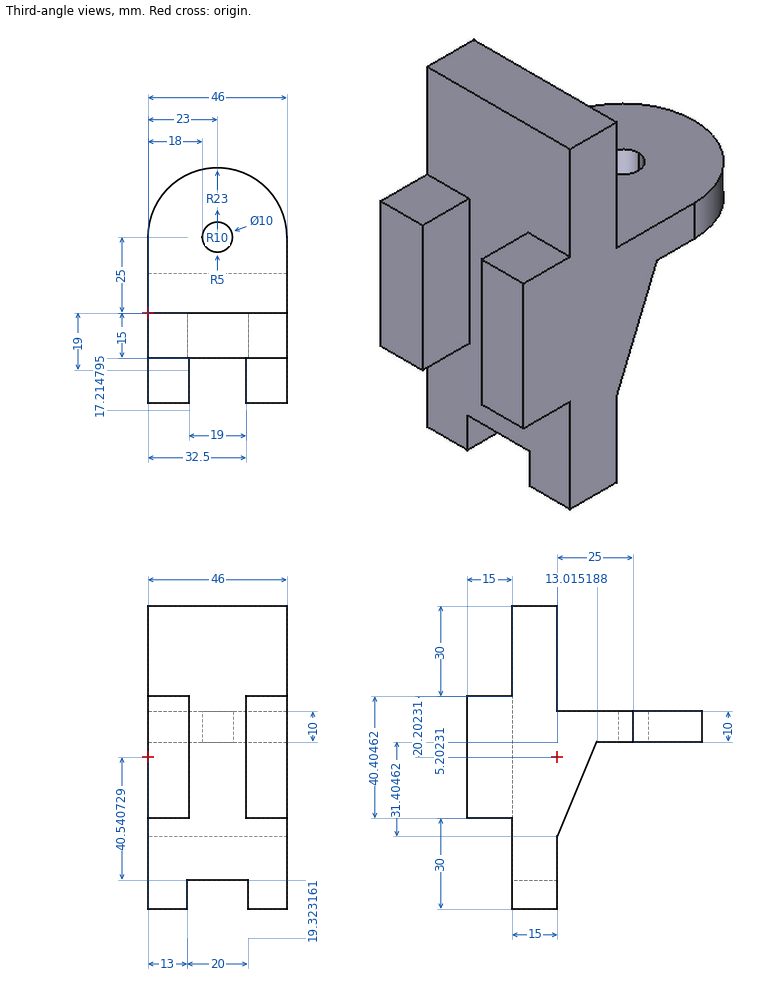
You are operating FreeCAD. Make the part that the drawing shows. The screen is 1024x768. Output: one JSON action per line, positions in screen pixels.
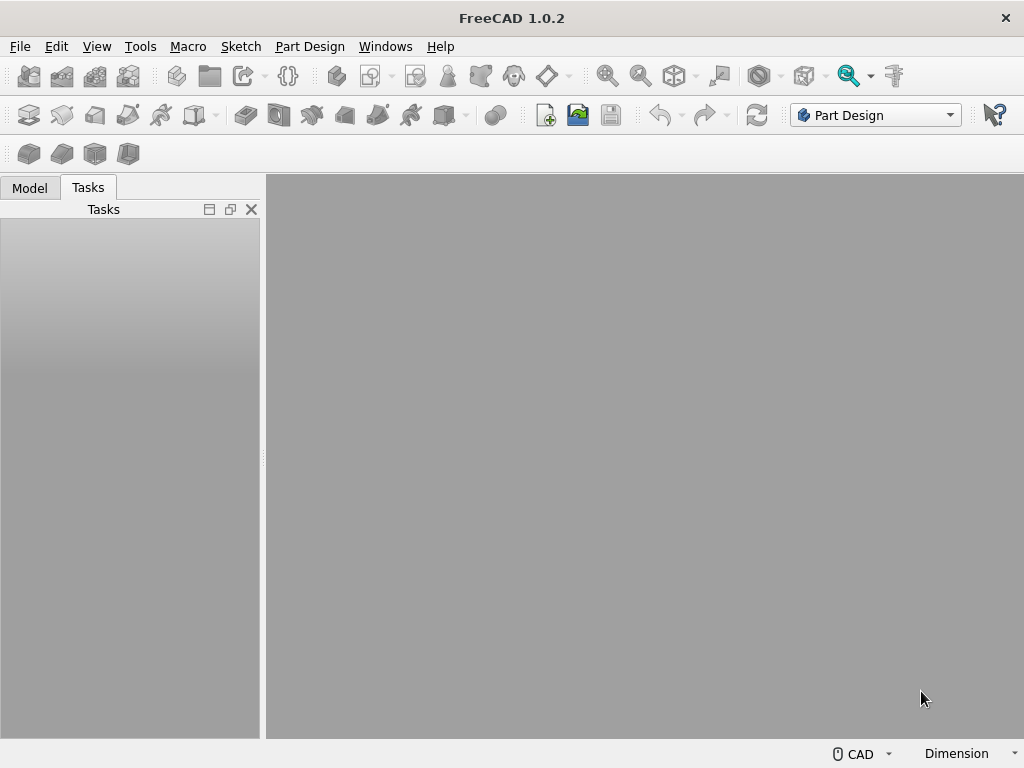
{"action": "left_click", "coordinate": [545, 116]}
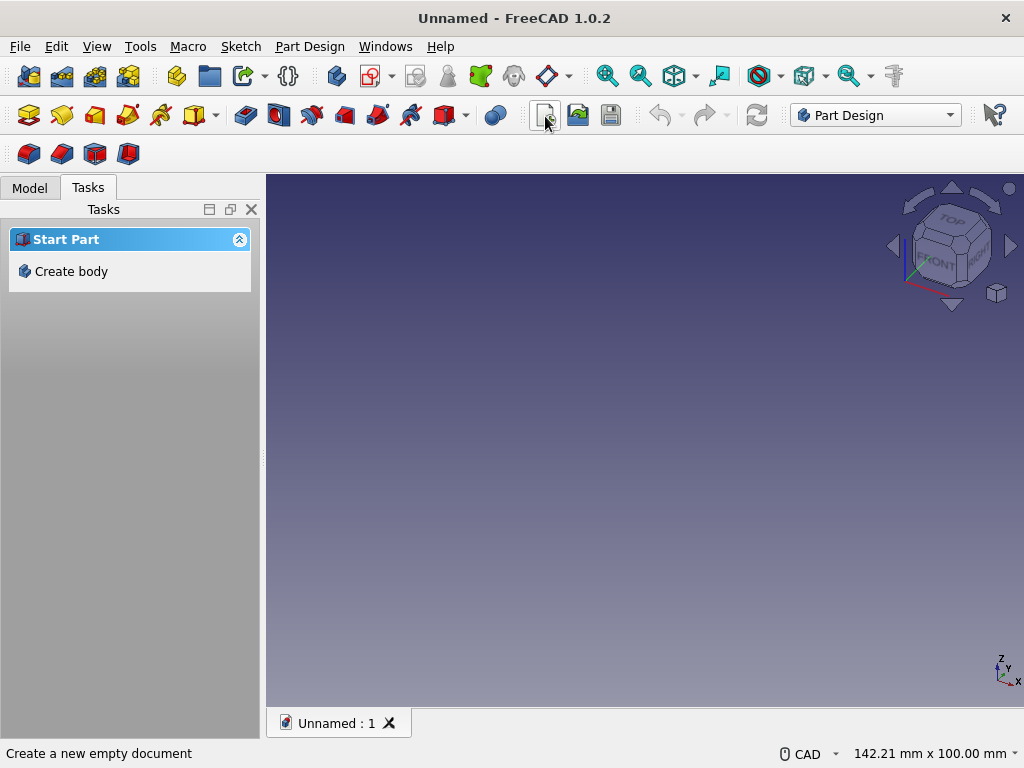
{"action": "left_click", "coordinate": [370, 76]}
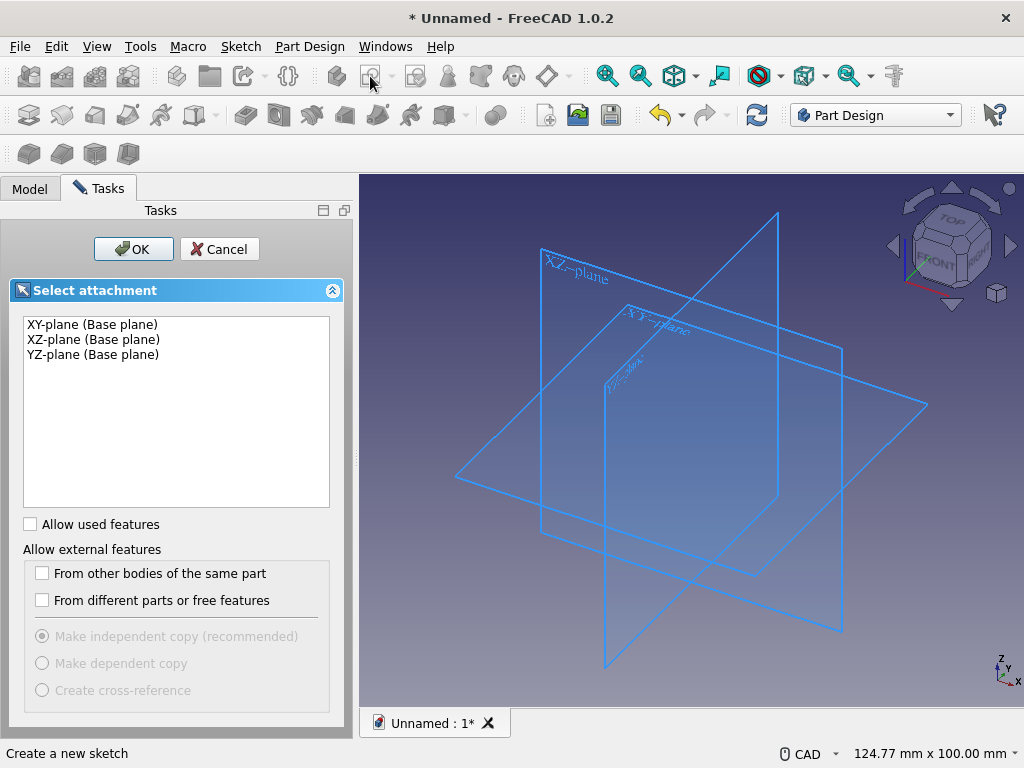
{"action": "left_click", "coordinate": [84, 354]}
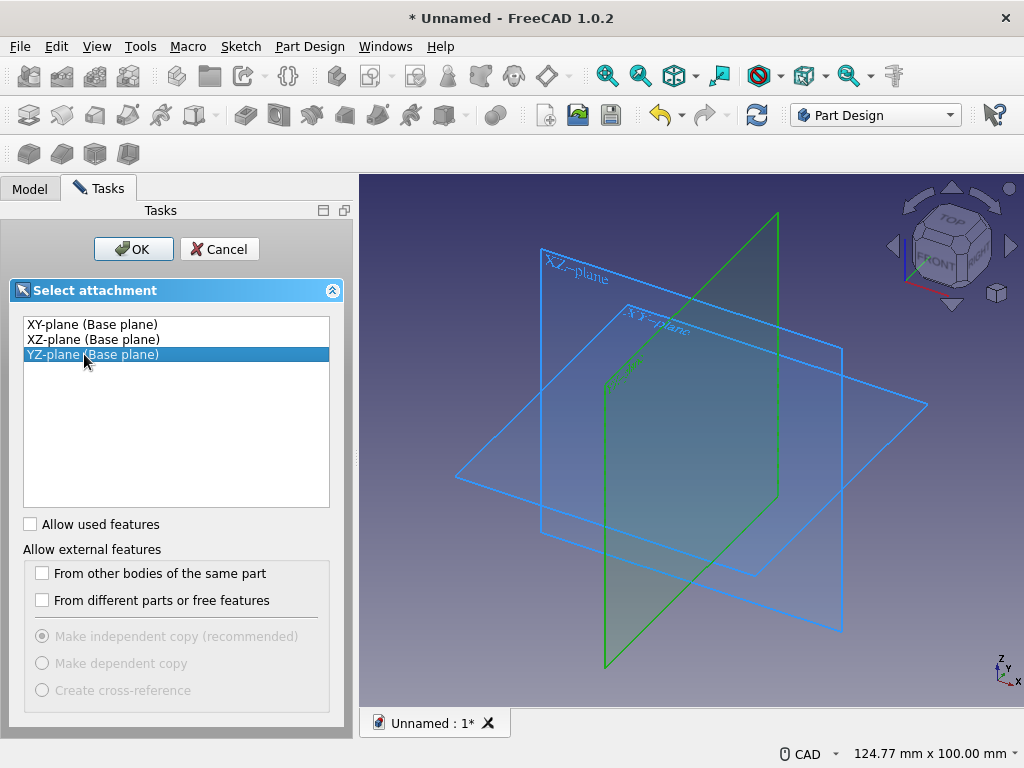
{"action": "left_click", "coordinate": [134, 249]}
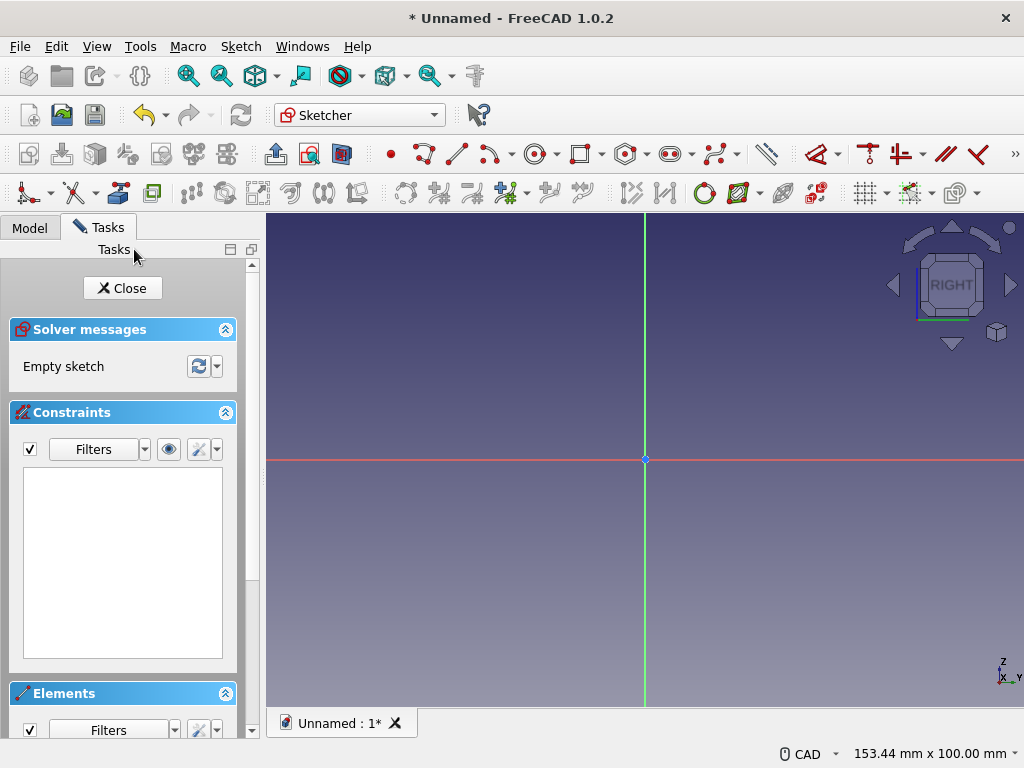
{"action": "scroll", "coordinate": [588, 460], "scroll_direction": "down", "scroll_amount": 2}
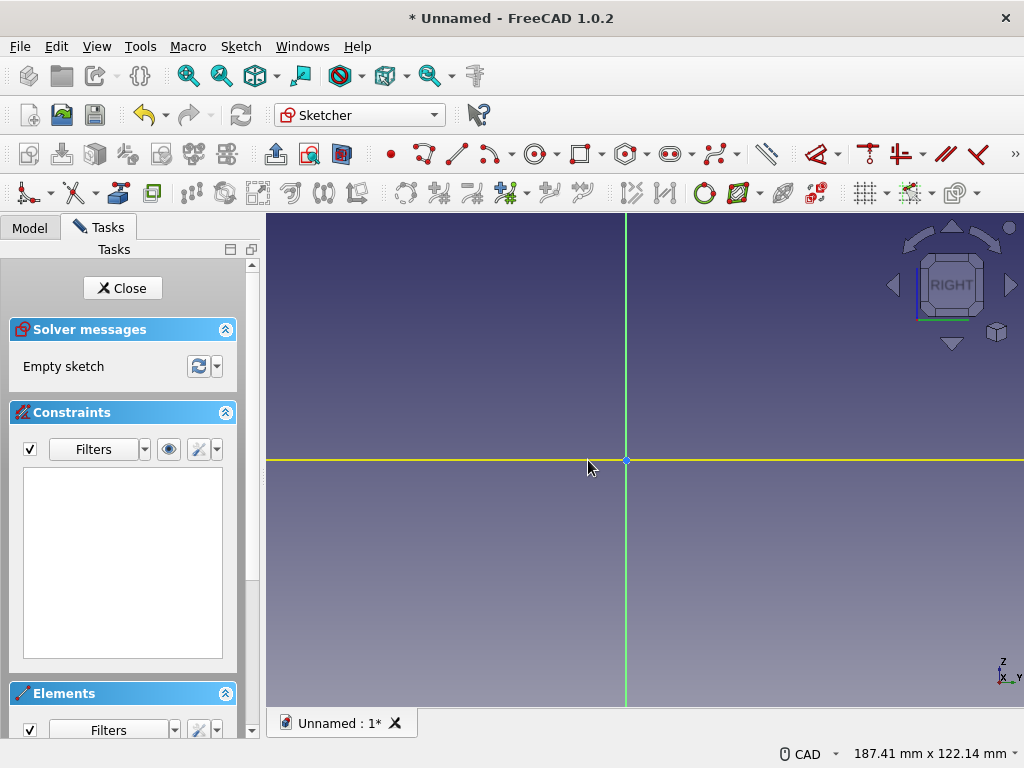
{"action": "left_click", "coordinate": [424, 154]}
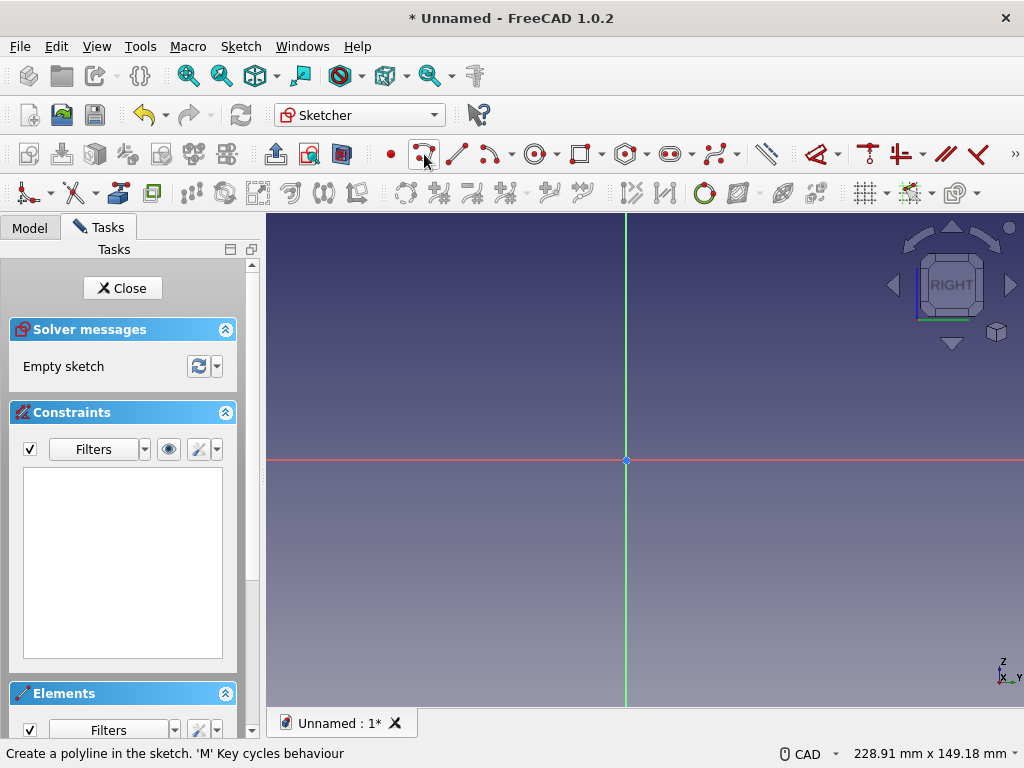
{"action": "left_click", "coordinate": [577, 393]}
{"action": "left_click", "coordinate": [527, 393]}
{"action": "left_click", "coordinate": [527, 527]}
{"action": "left_click", "coordinate": [577, 527]}
{"action": "left_click", "coordinate": [577, 626]}
{"action": "left_click", "coordinate": [626, 626]}
{"action": "left_click", "coordinate": [617, 294]}
{"action": "left_click", "coordinate": [577, 294]}
{"action": "left_click", "coordinate": [577, 394]}
{"action": "key", "text": "Escape"}
{"action": "key", "text": "Escape"}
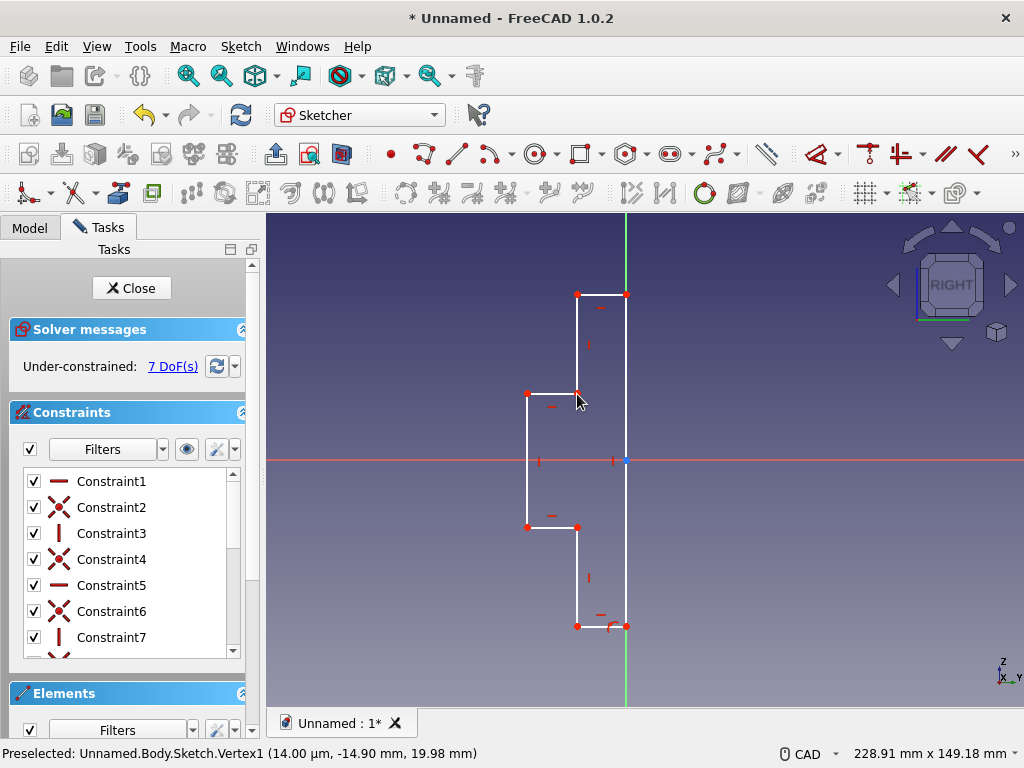
{"action": "left_click", "coordinate": [816, 154]}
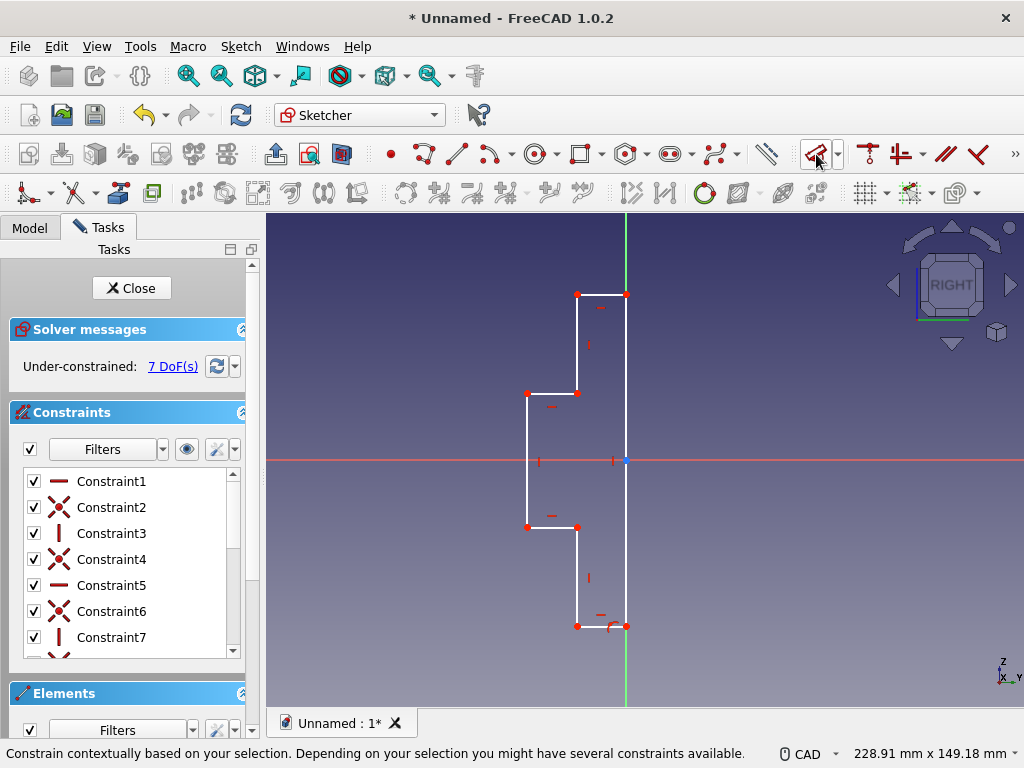
{"action": "left_click", "coordinate": [562, 394]}
{"action": "left_click", "coordinate": [552, 360]}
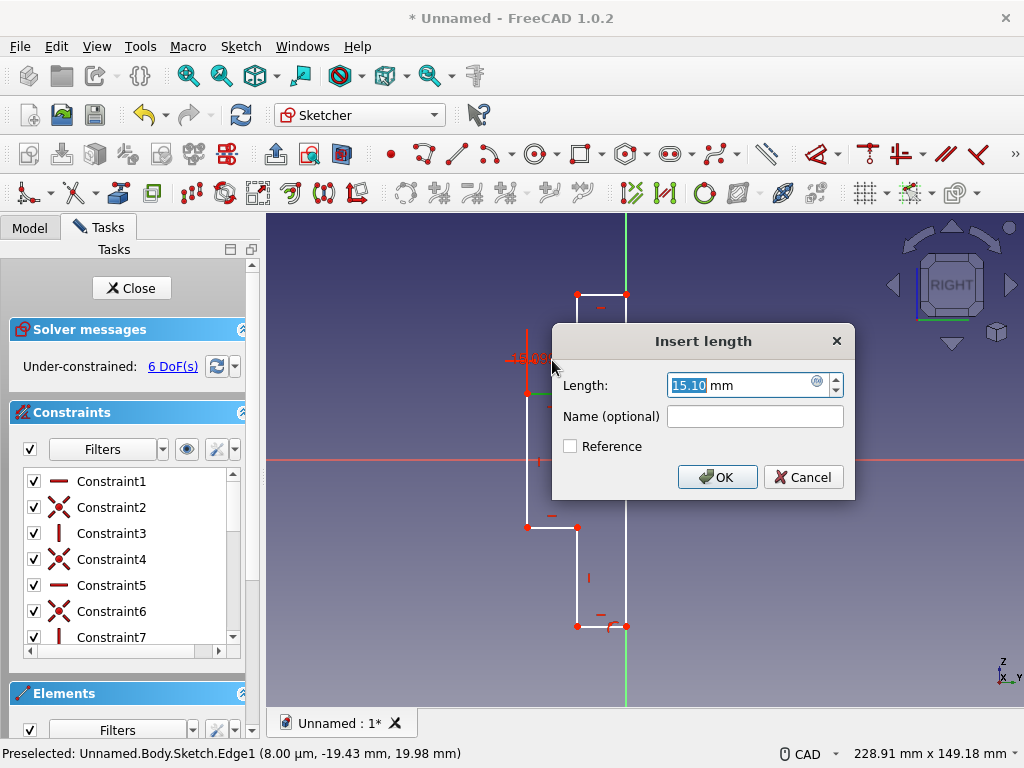
{"action": "type", "text": "15"}
{"action": "key", "text": "Return"}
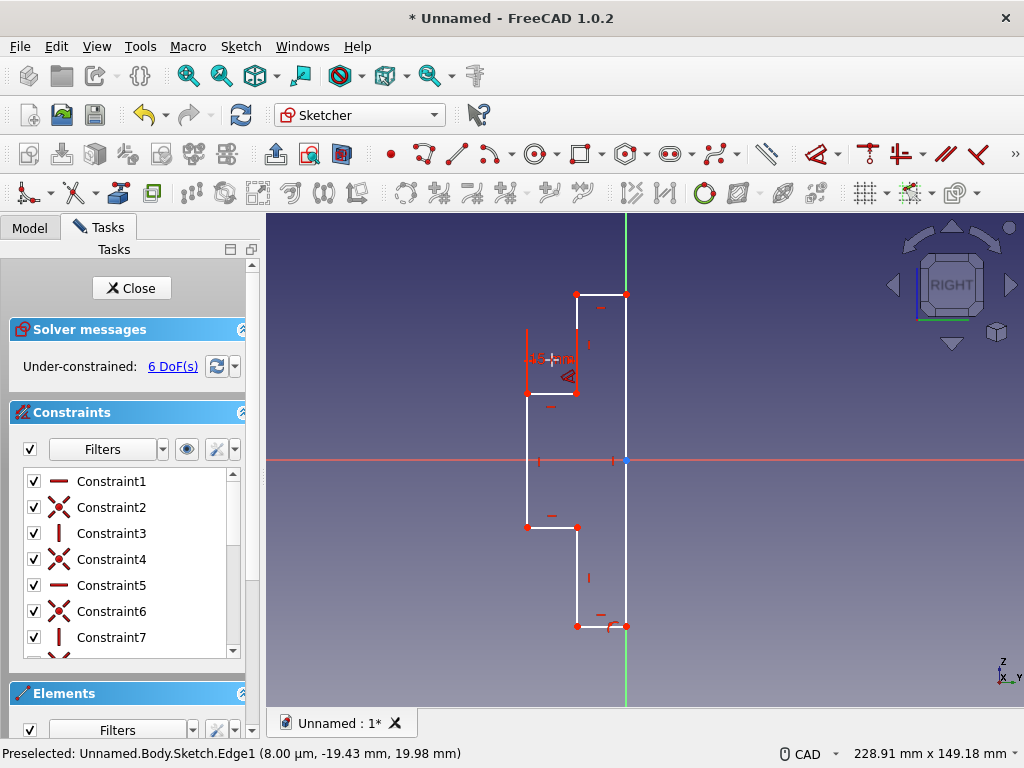
{"action": "left_click", "coordinate": [542, 528]}
{"action": "left_click", "coordinate": [552, 562]}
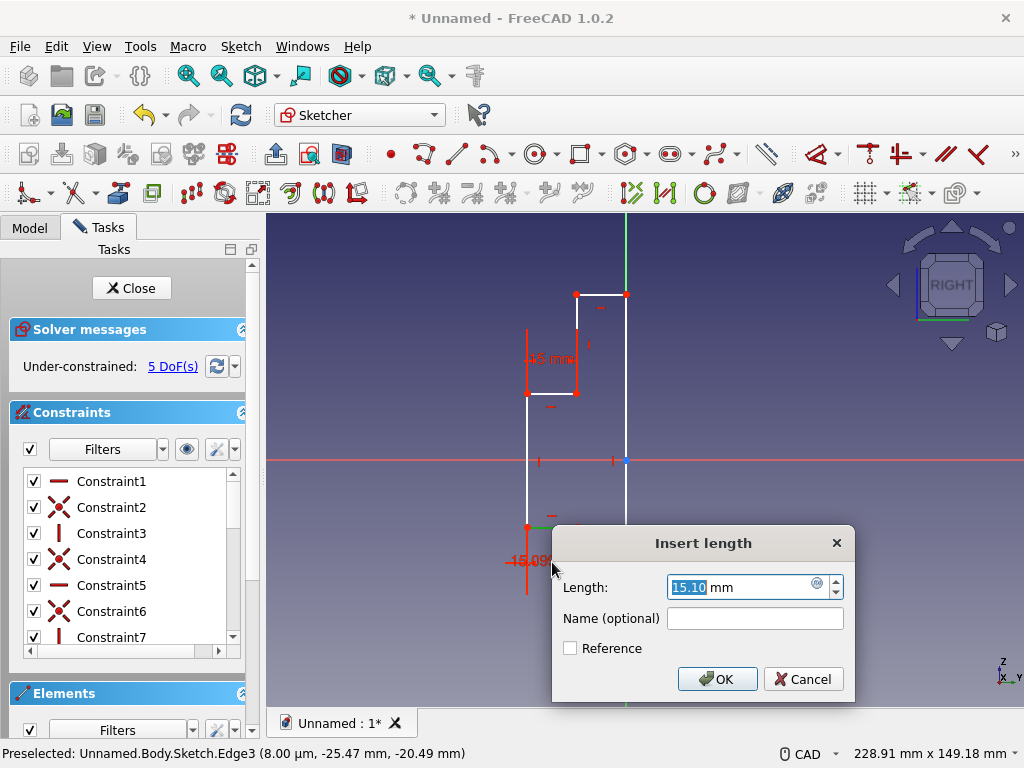
{"action": "type", "text": "15"}
{"action": "key", "text": "Return"}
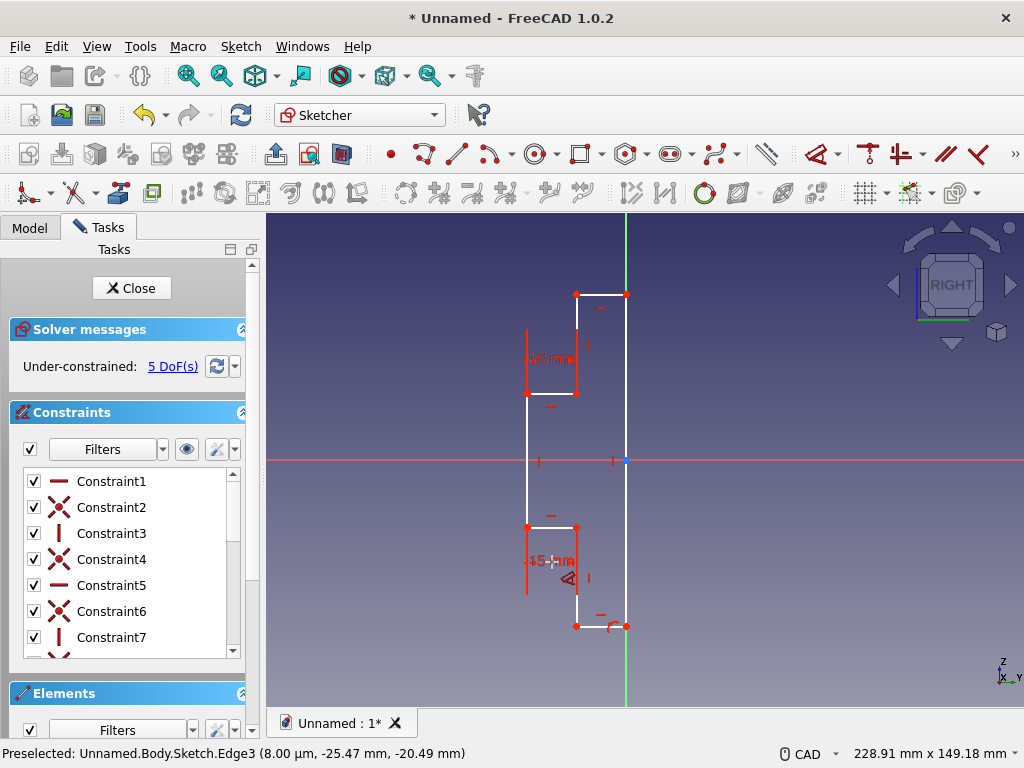
{"action": "left_click", "coordinate": [577, 558]}
{"action": "left_click", "coordinate": [543, 600]}